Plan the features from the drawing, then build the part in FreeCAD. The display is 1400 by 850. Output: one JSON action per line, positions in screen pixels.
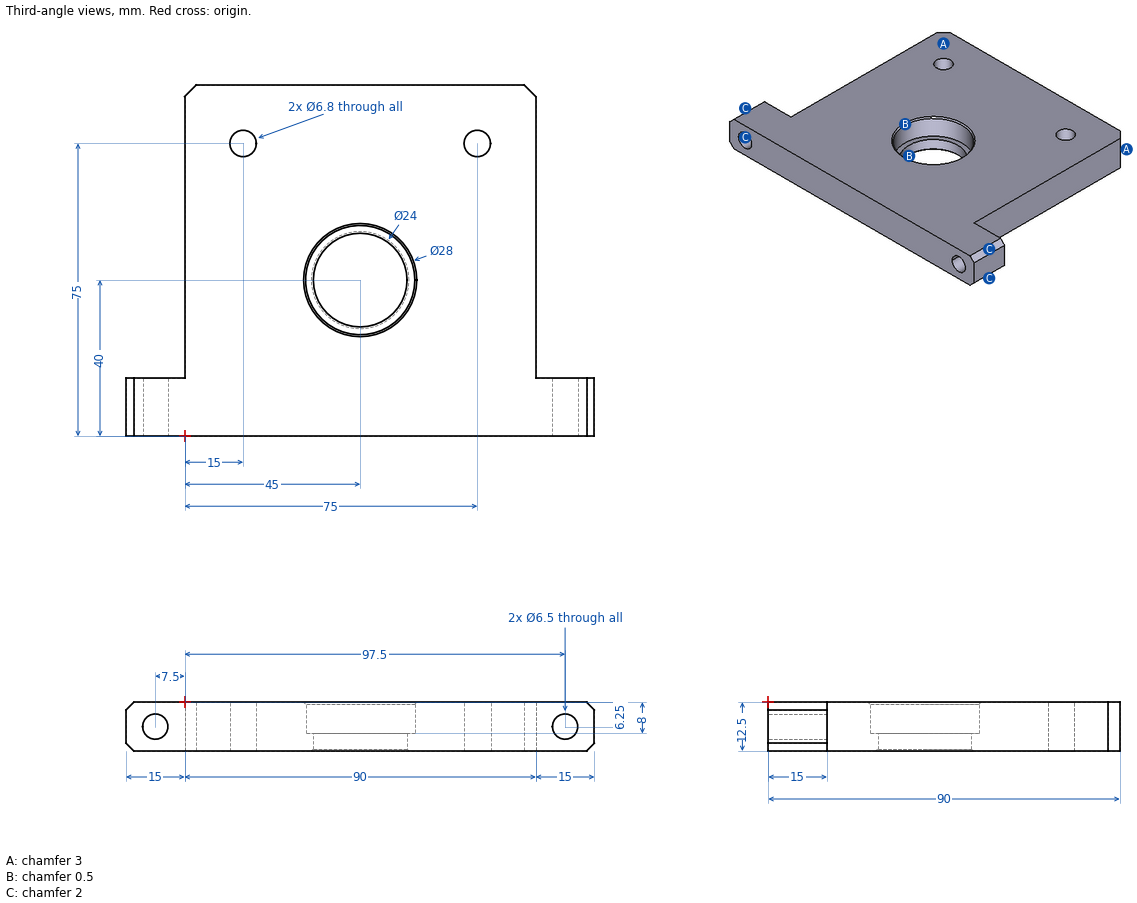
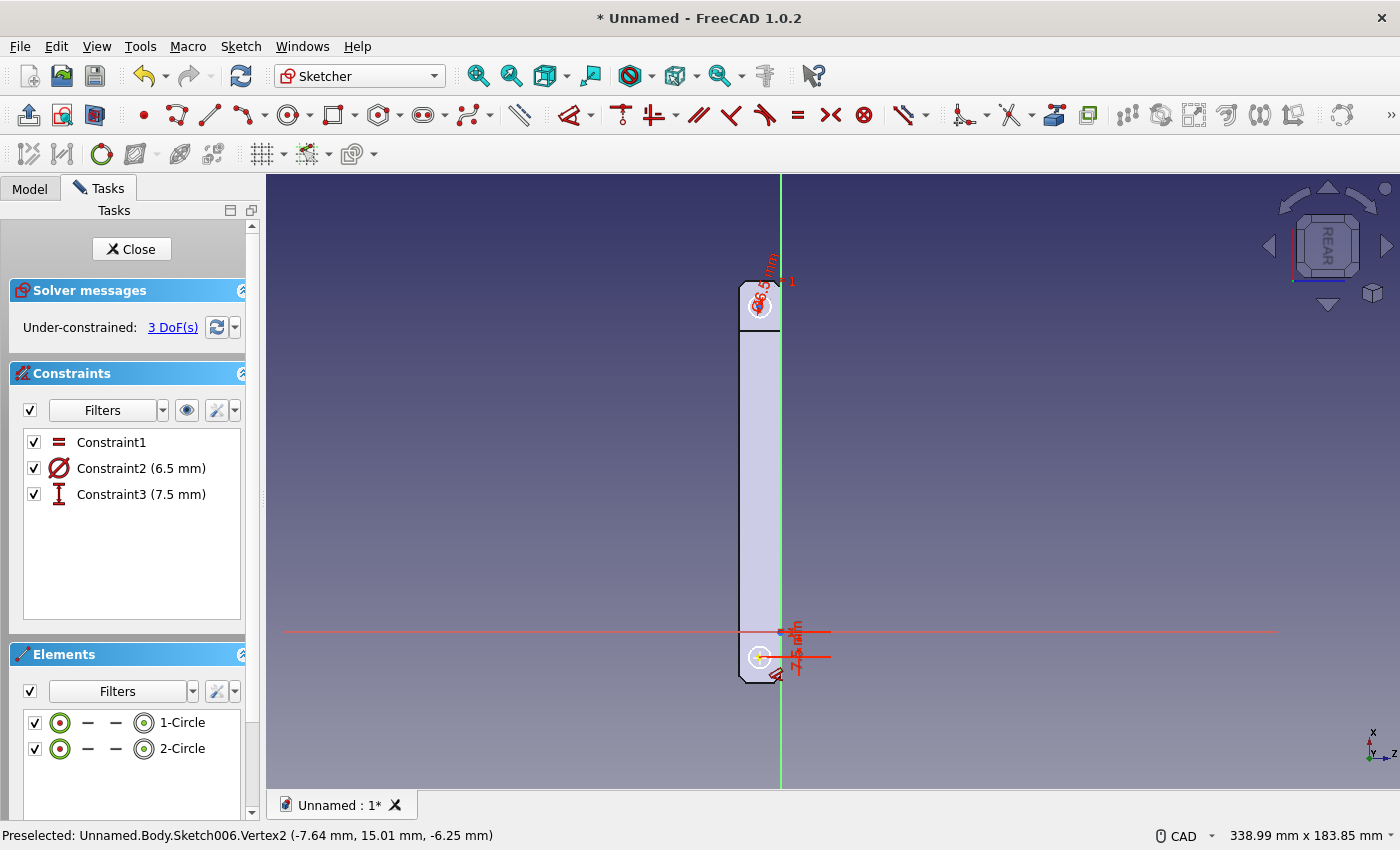
{"action": "scroll", "coordinate": [760, 307], "scroll_direction": "up", "scroll_amount": 4}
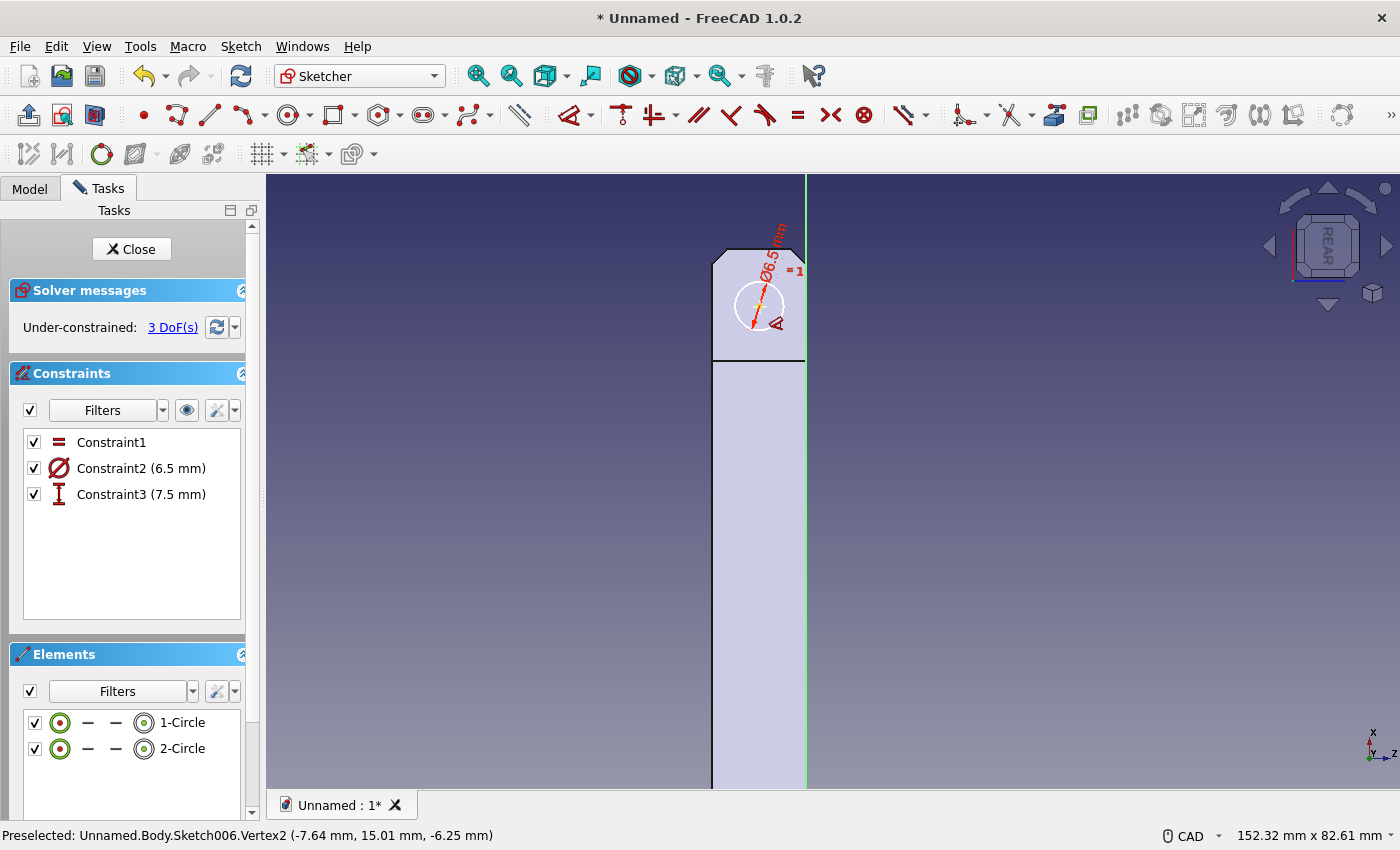
{"action": "left_click", "coordinate": [759, 306]}
{"action": "left_click", "coordinate": [782, 224]}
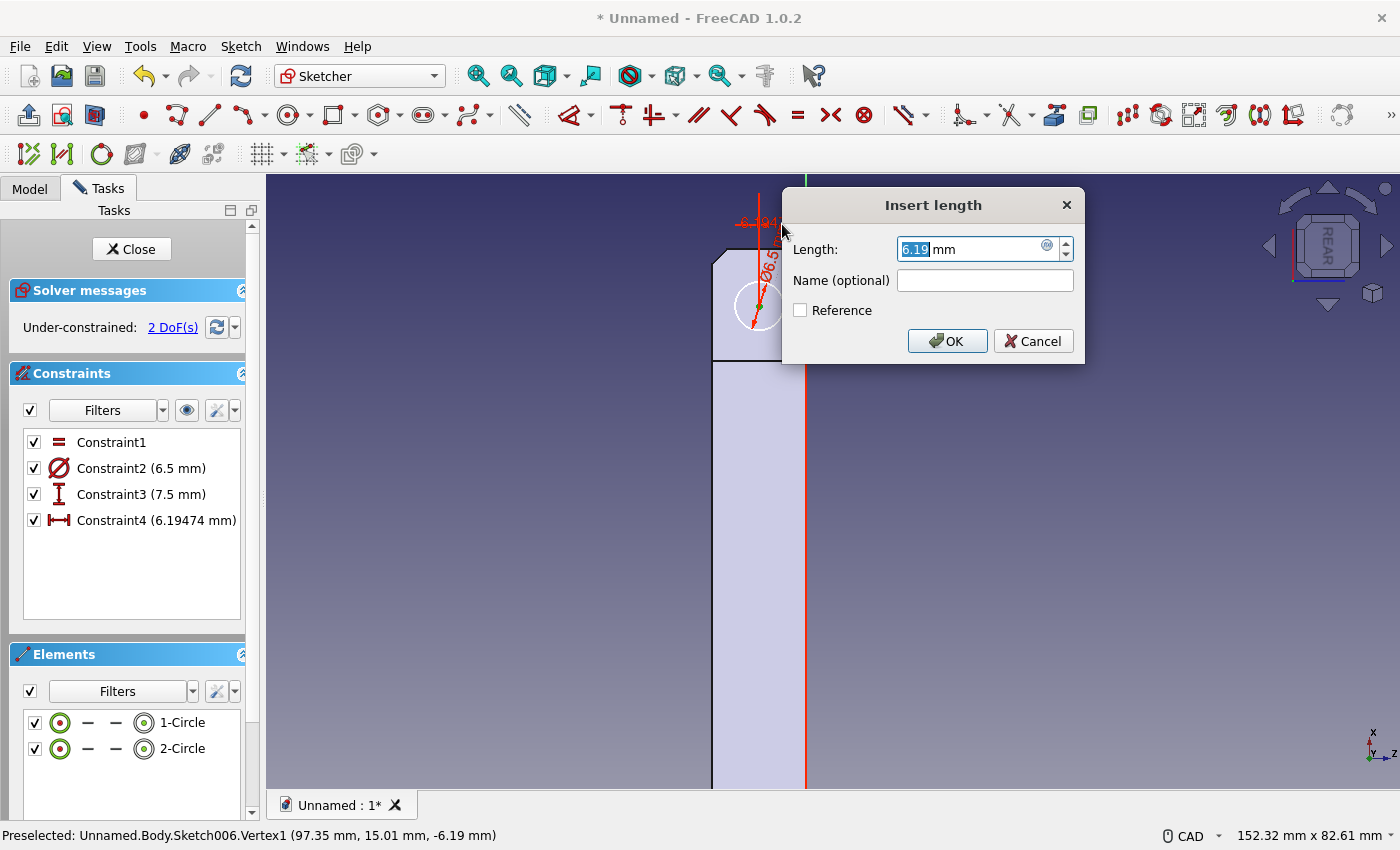
{"action": "type", "text": "6.25"}
{"action": "key", "text": "Return"}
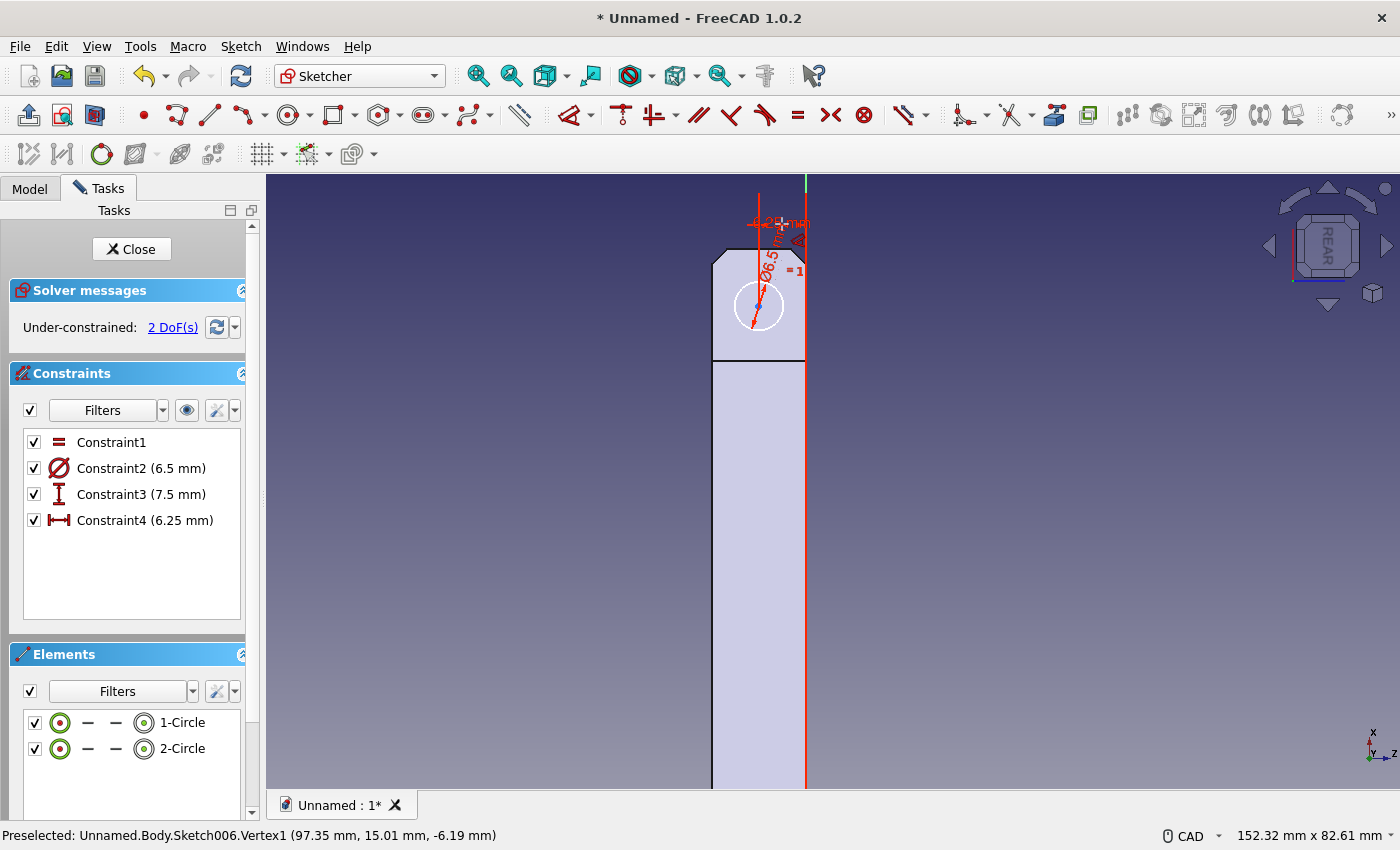
{"action": "left_click", "coordinate": [759, 306]}
{"action": "left_click", "coordinate": [840, 534]}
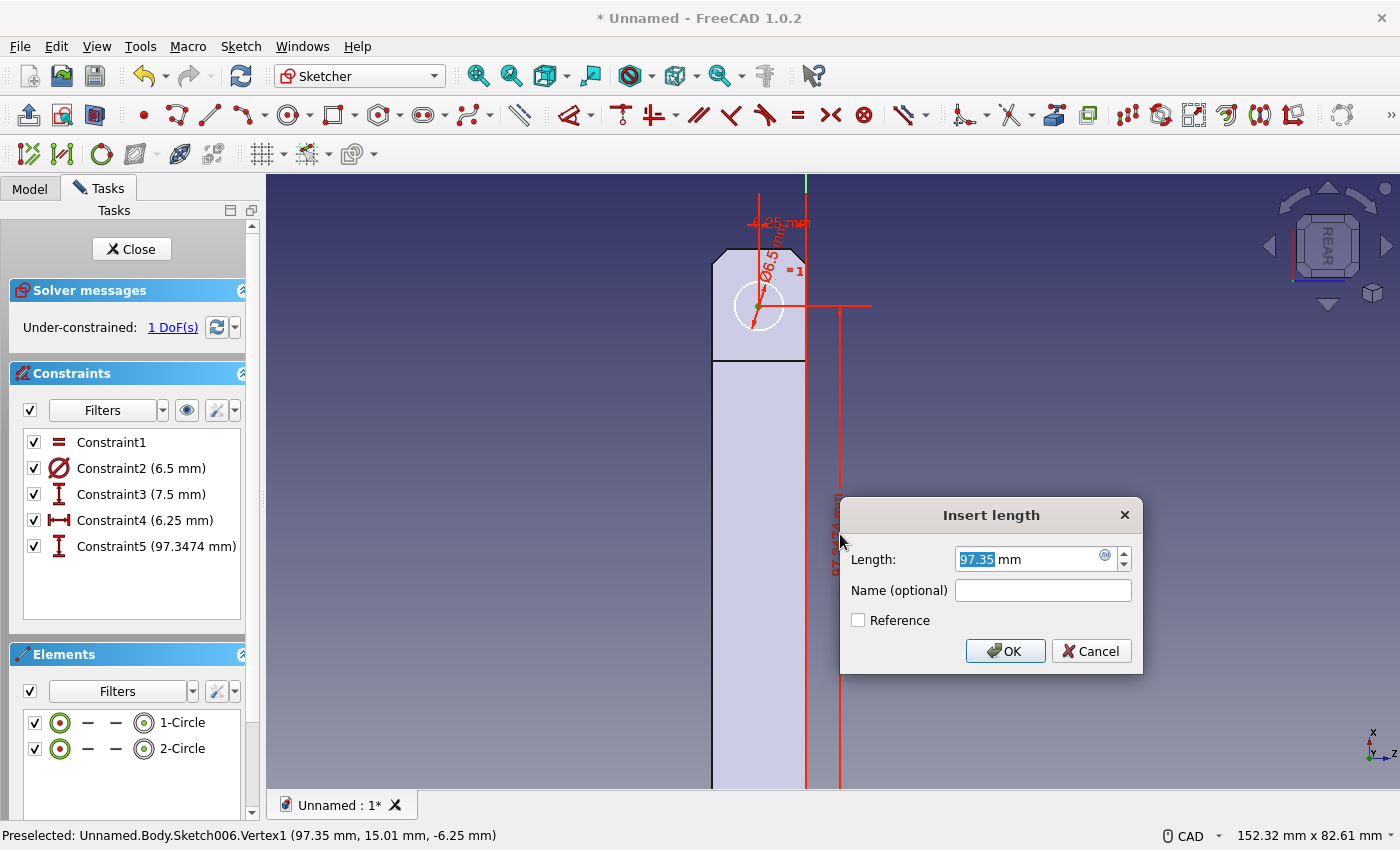
{"action": "type", "text": "97.5"}
{"action": "key", "text": "Return"}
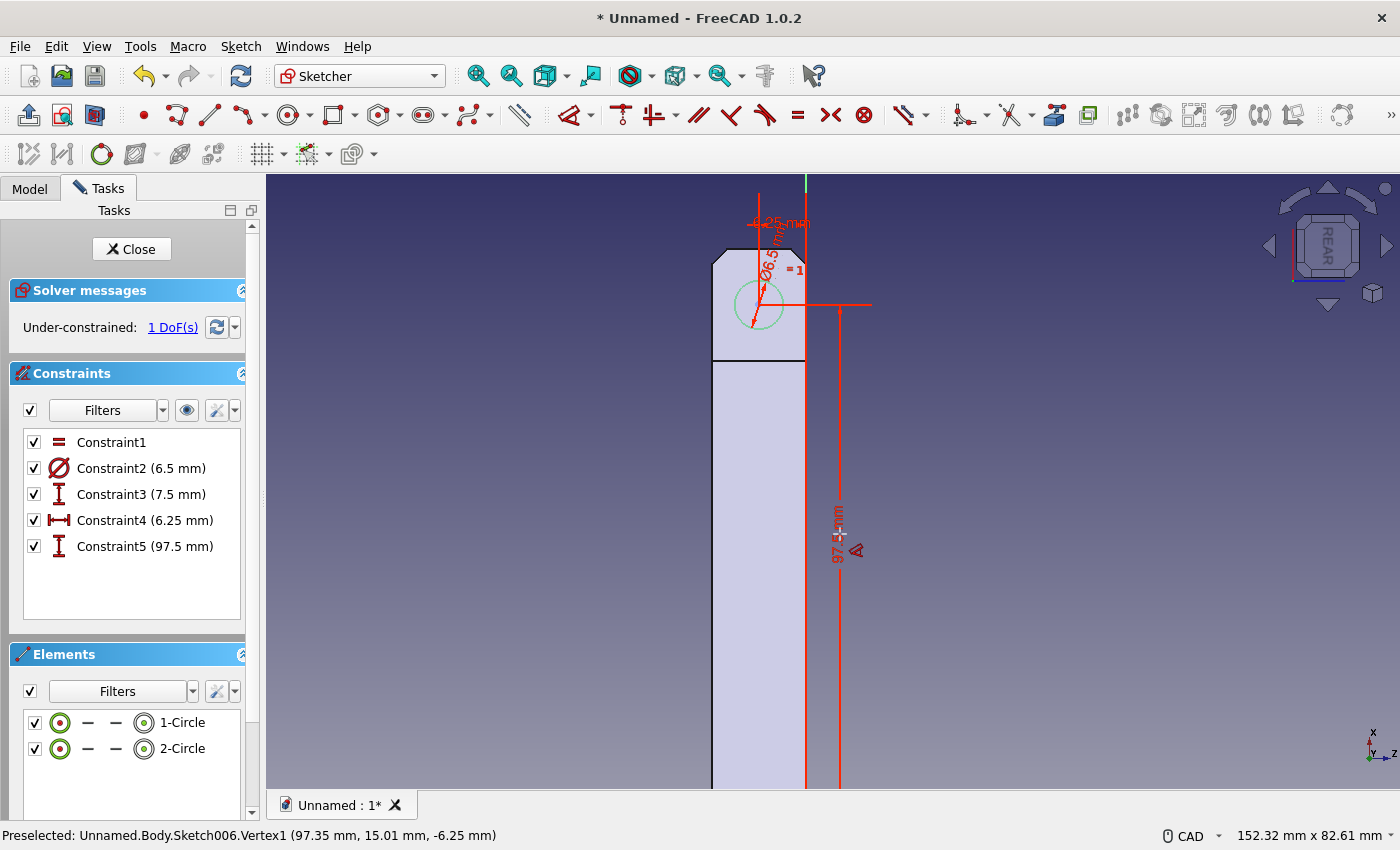
{"action": "scroll", "coordinate": [760, 307], "scroll_direction": "down", "scroll_amount": 4}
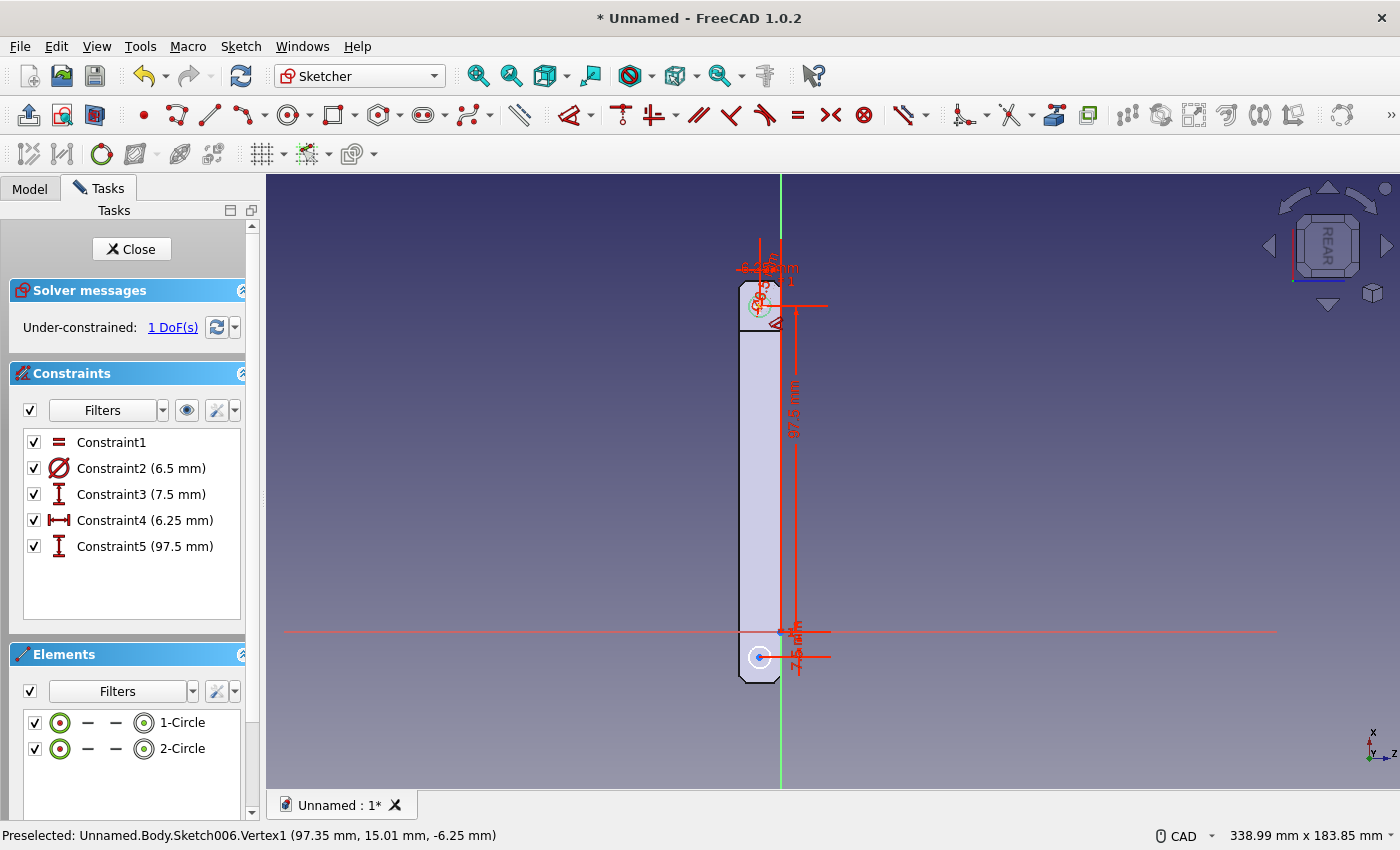
{"action": "scroll", "coordinate": [760, 657], "scroll_direction": "up", "scroll_amount": 4}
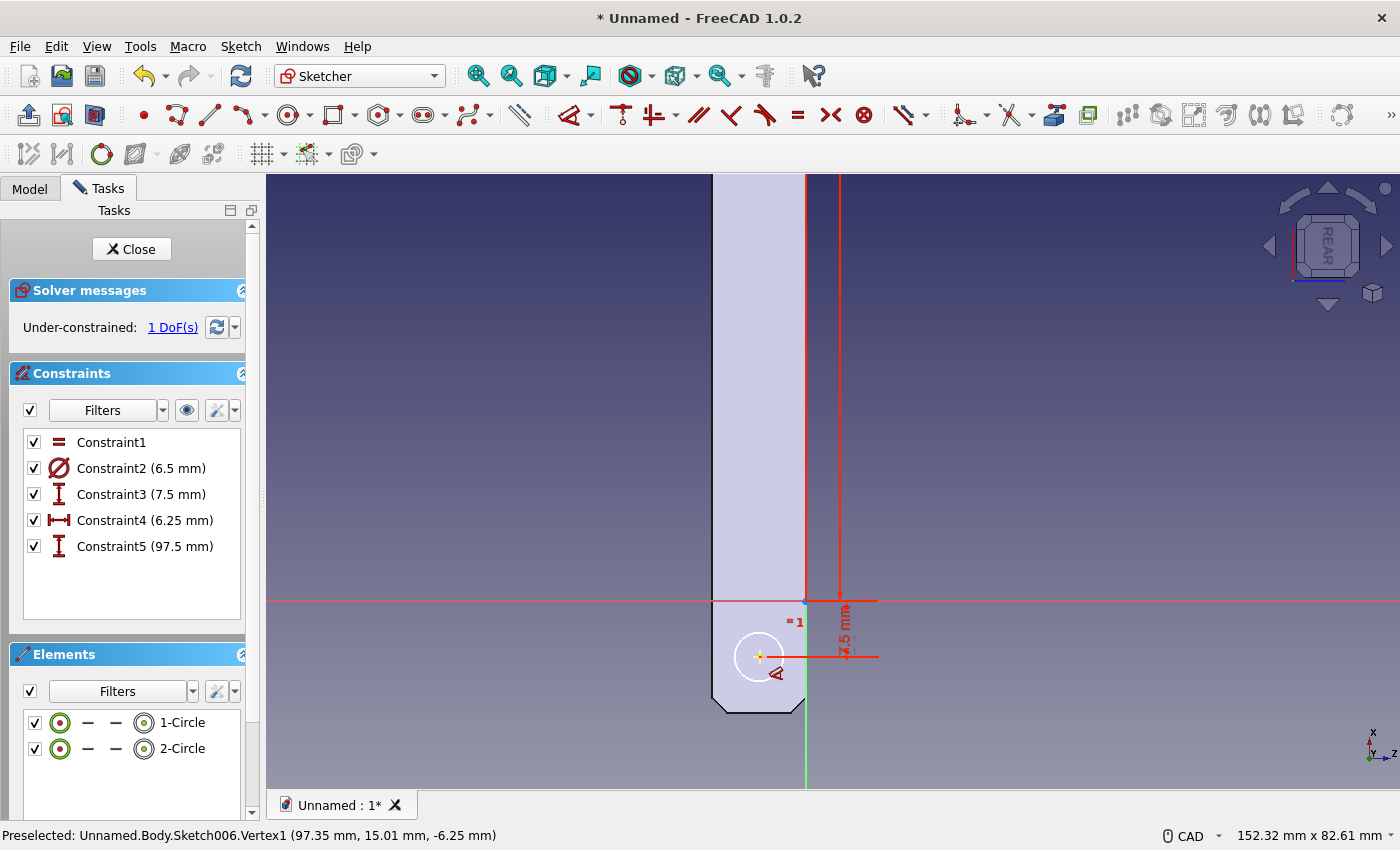
{"action": "left_click", "coordinate": [759, 657]}
{"action": "left_click", "coordinate": [782, 691]}